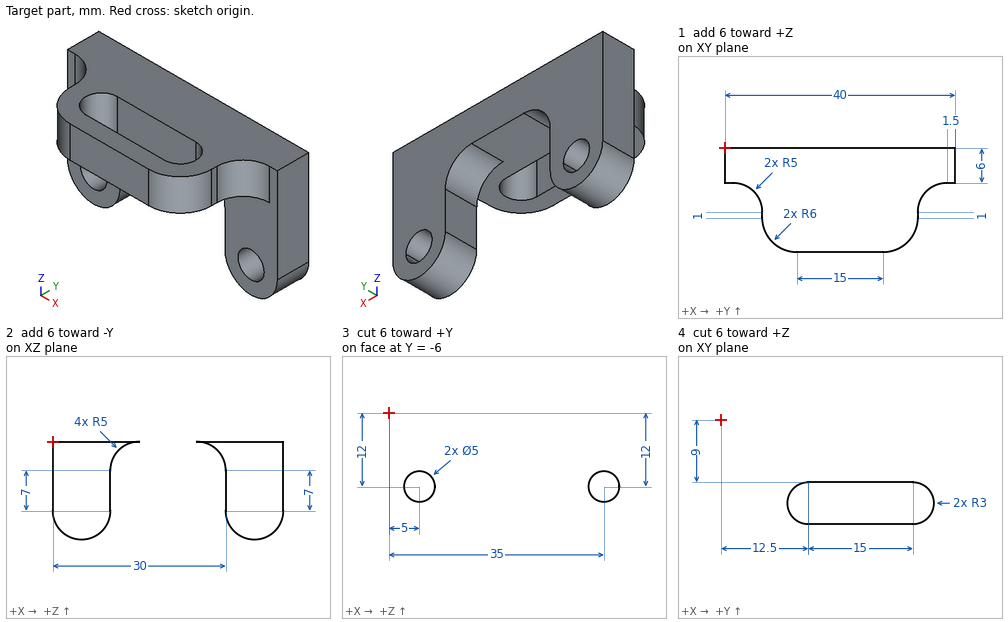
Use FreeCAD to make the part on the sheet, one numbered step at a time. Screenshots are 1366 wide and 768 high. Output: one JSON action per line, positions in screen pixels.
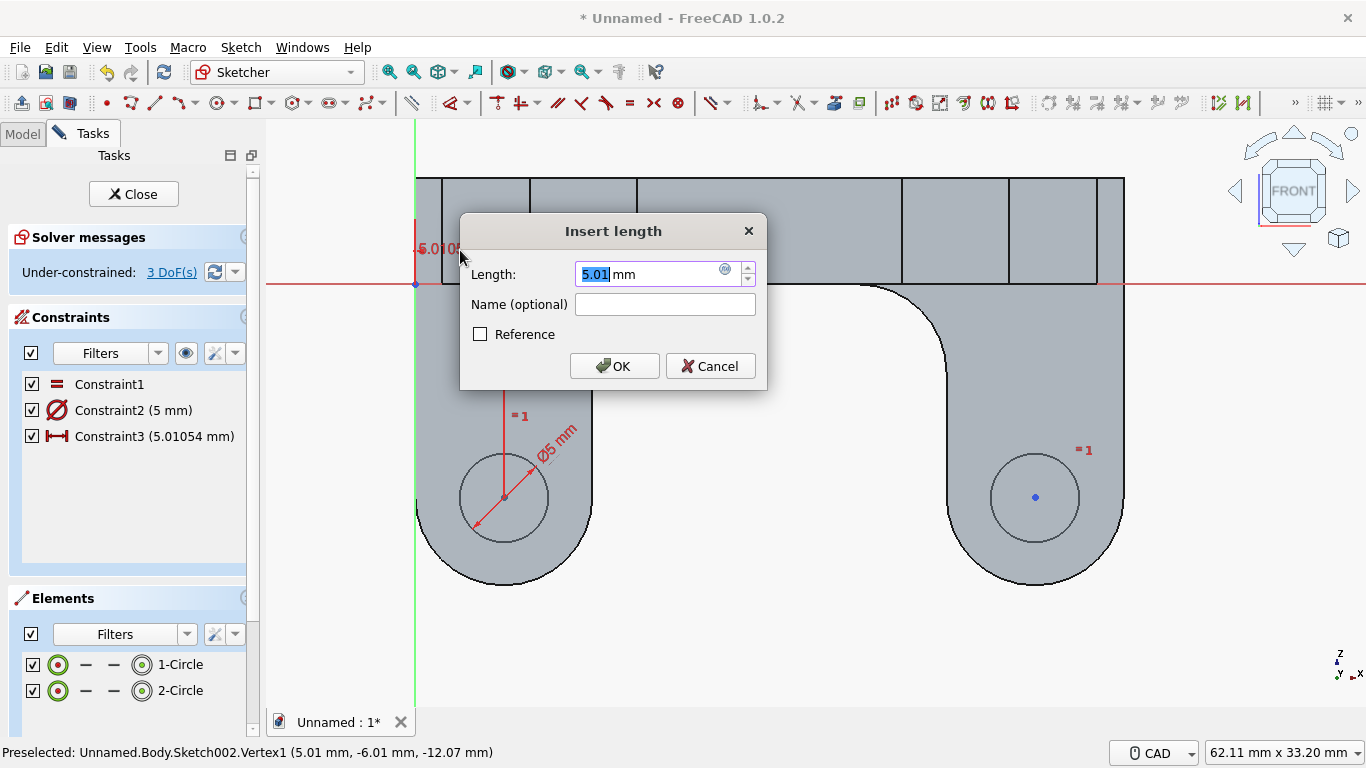
{"action": "type", "text": "5"}
{"action": "key", "text": "Return"}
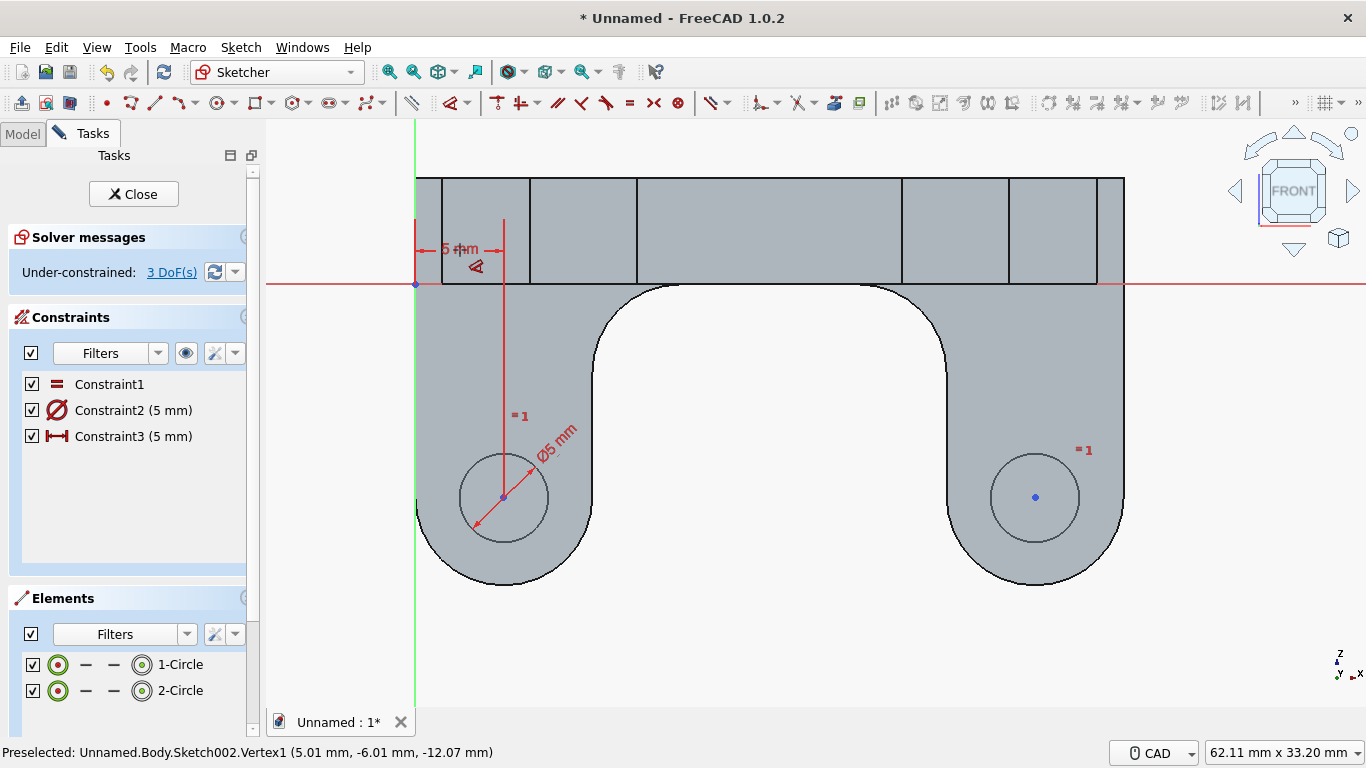
{"action": "left_click", "coordinate": [504, 498]}
{"action": "left_click", "coordinate": [381, 391]}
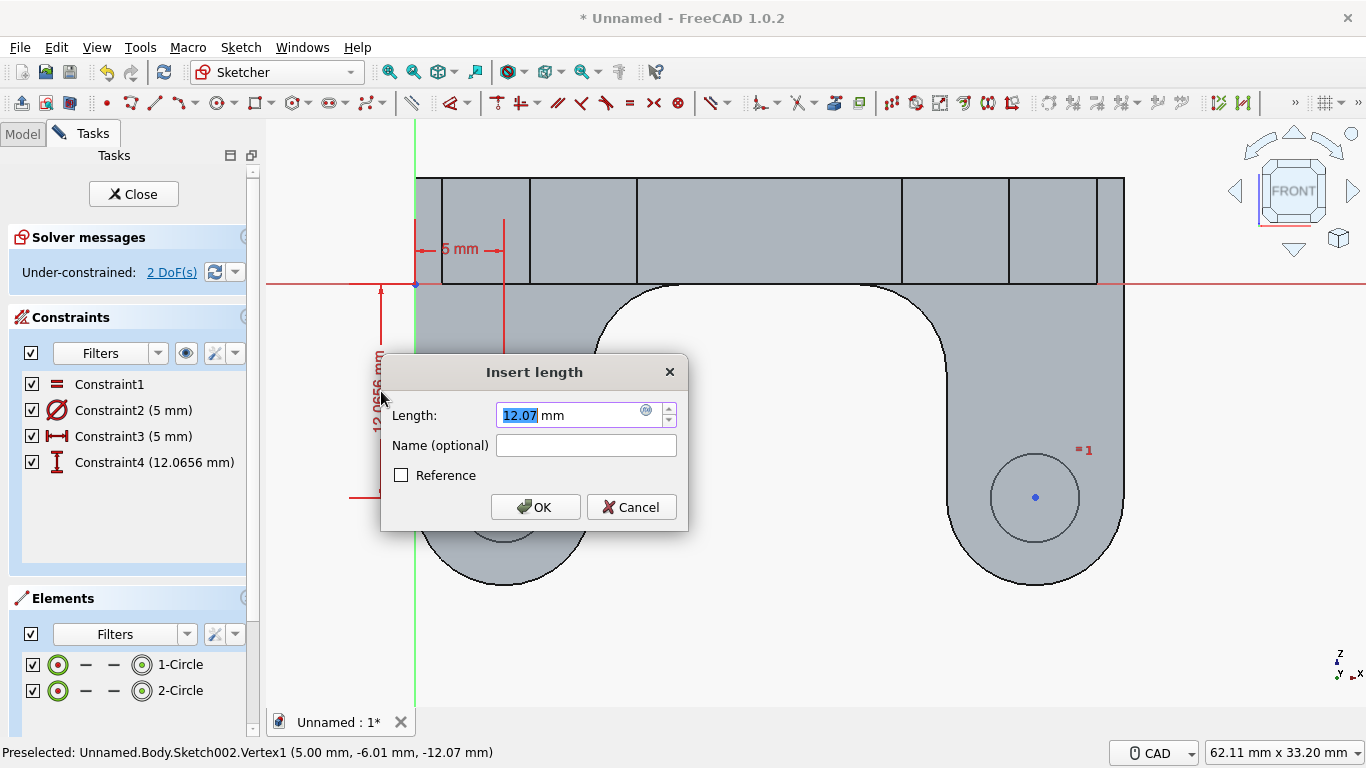
{"action": "type", "text": "12"}
{"action": "key", "text": "Return"}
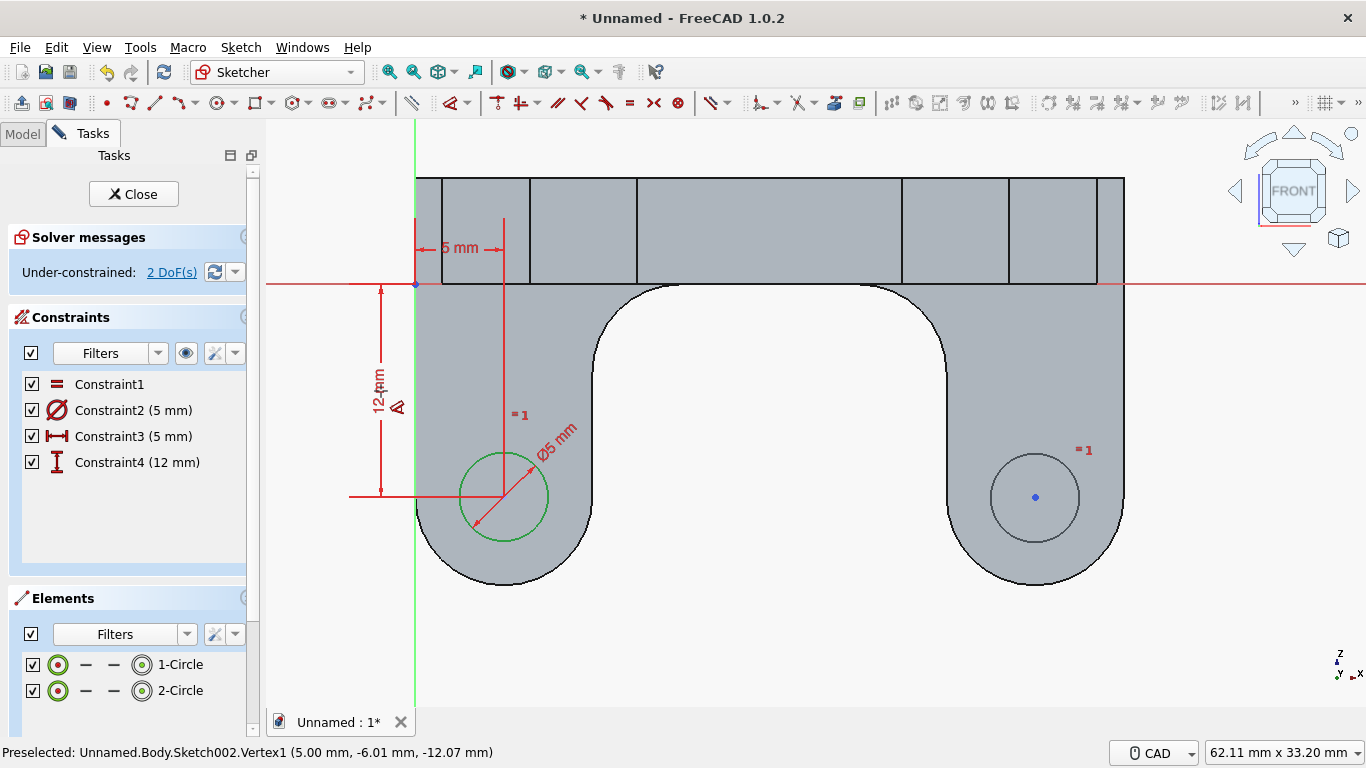
{"action": "left_click", "coordinate": [1035, 498]}
{"action": "left_click", "coordinate": [725, 250]}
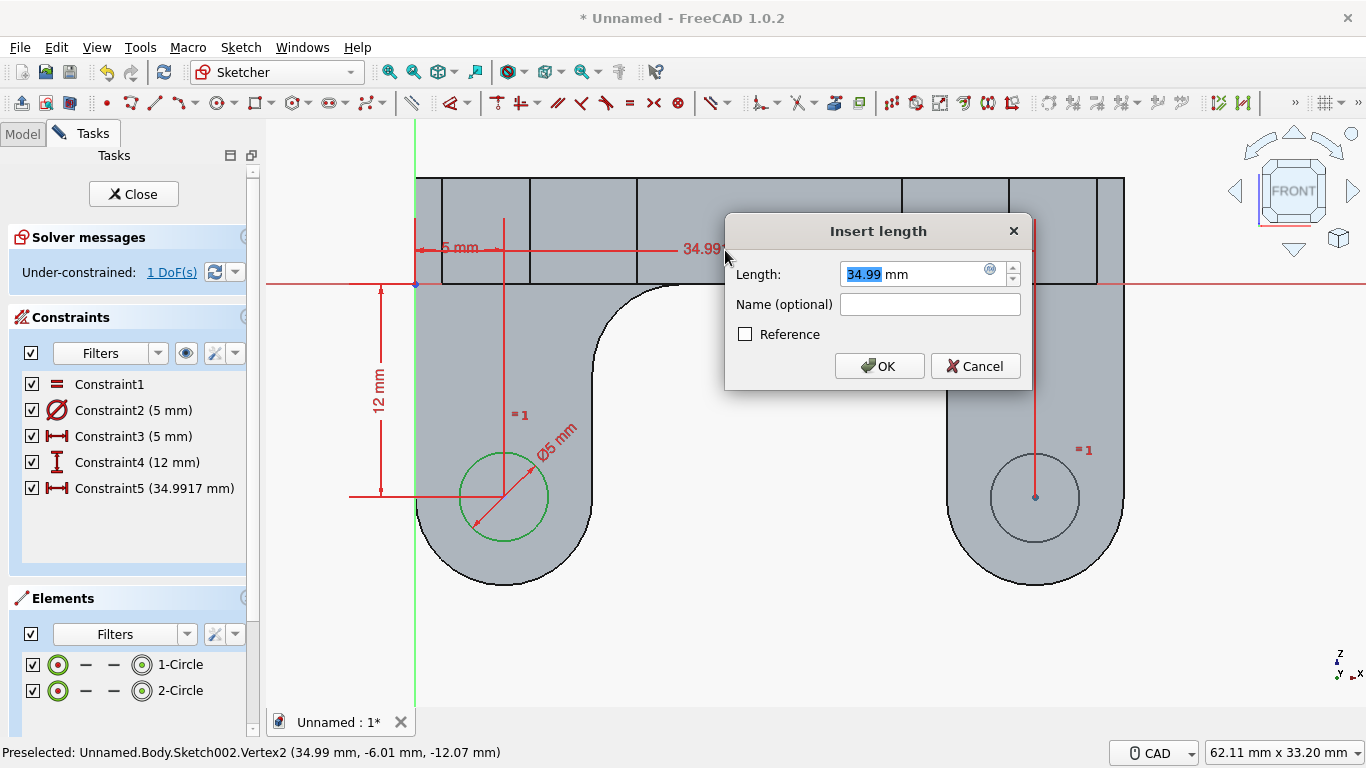
{"action": "type", "text": "35"}
{"action": "key", "text": "Return"}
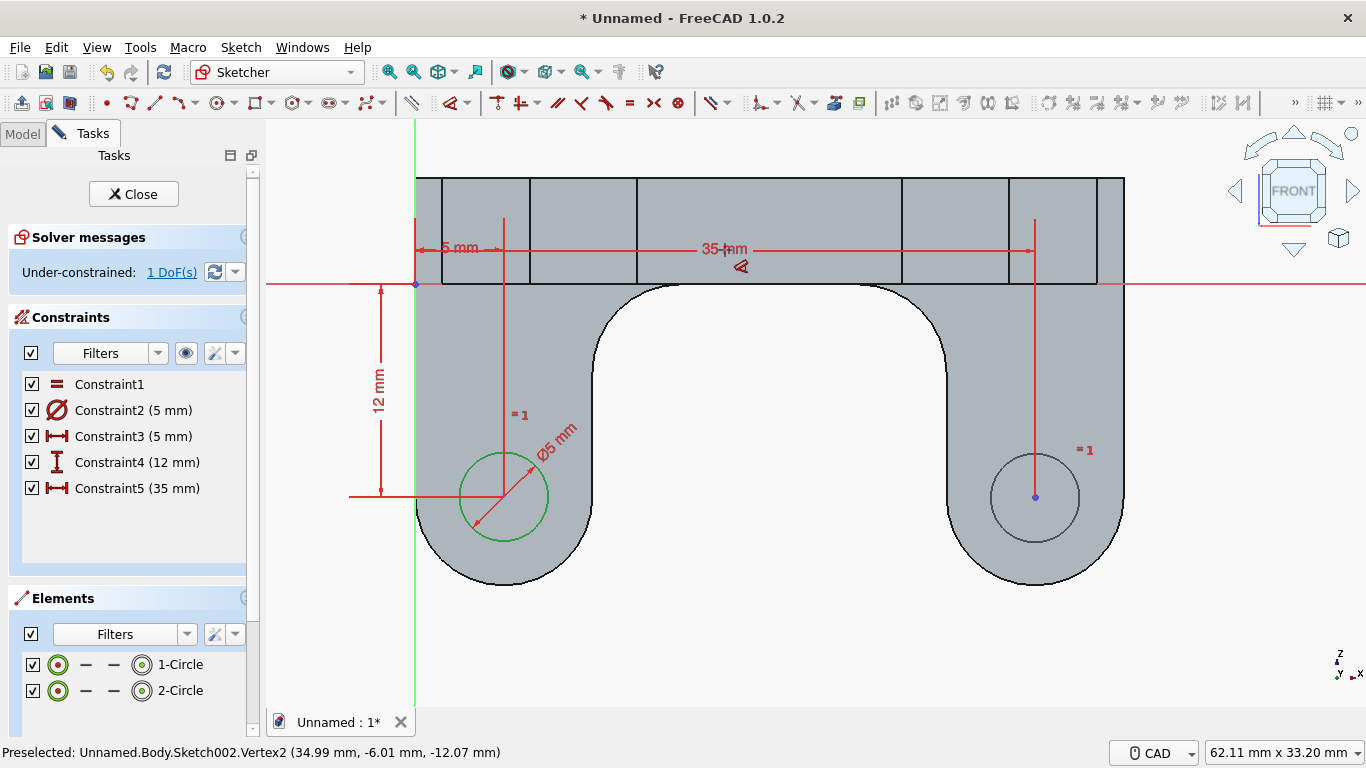
{"action": "left_click", "coordinate": [1035, 498]}
{"action": "left_click", "coordinate": [381, 342]}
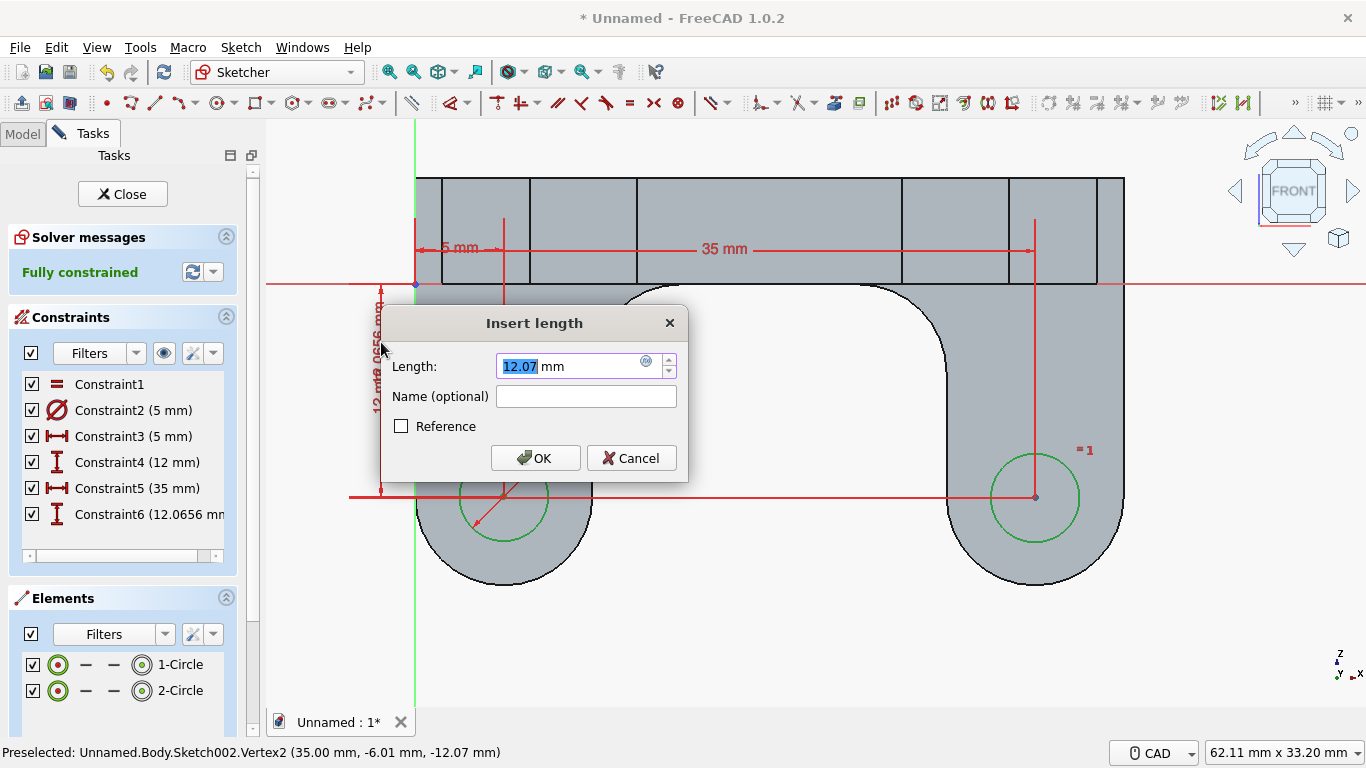
{"action": "type", "text": "12"}
{"action": "key", "text": "Return"}
{"action": "key", "text": "Escape"}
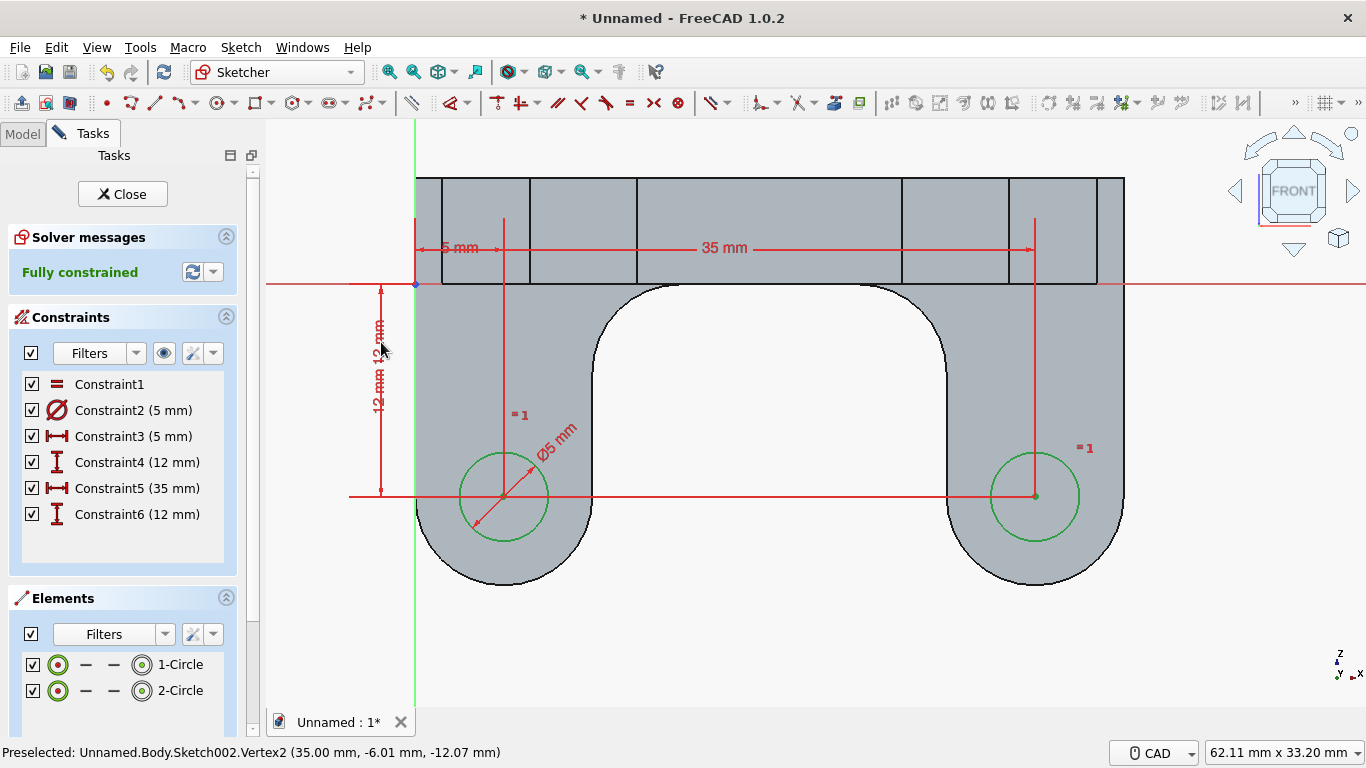
{"action": "left_click", "coordinate": [123, 194]}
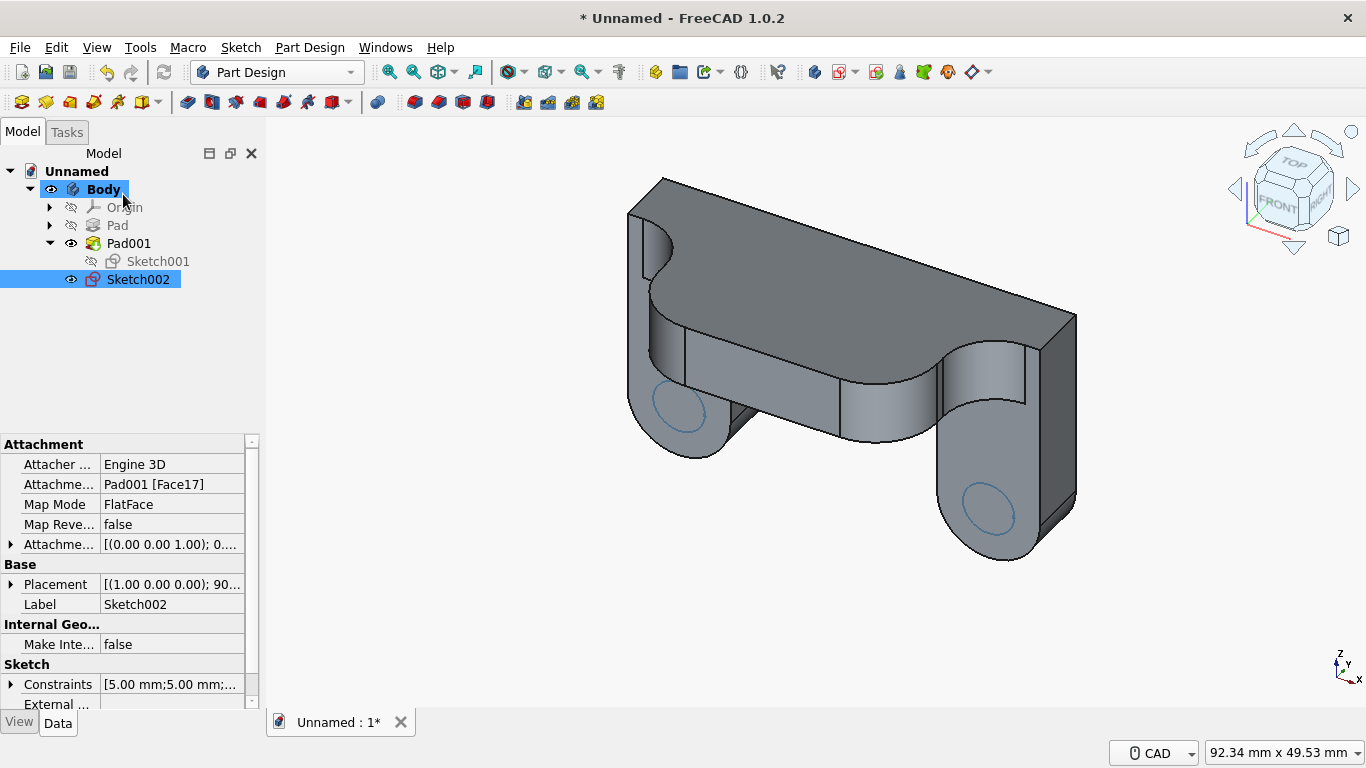
{"action": "left_click", "coordinate": [188, 102]}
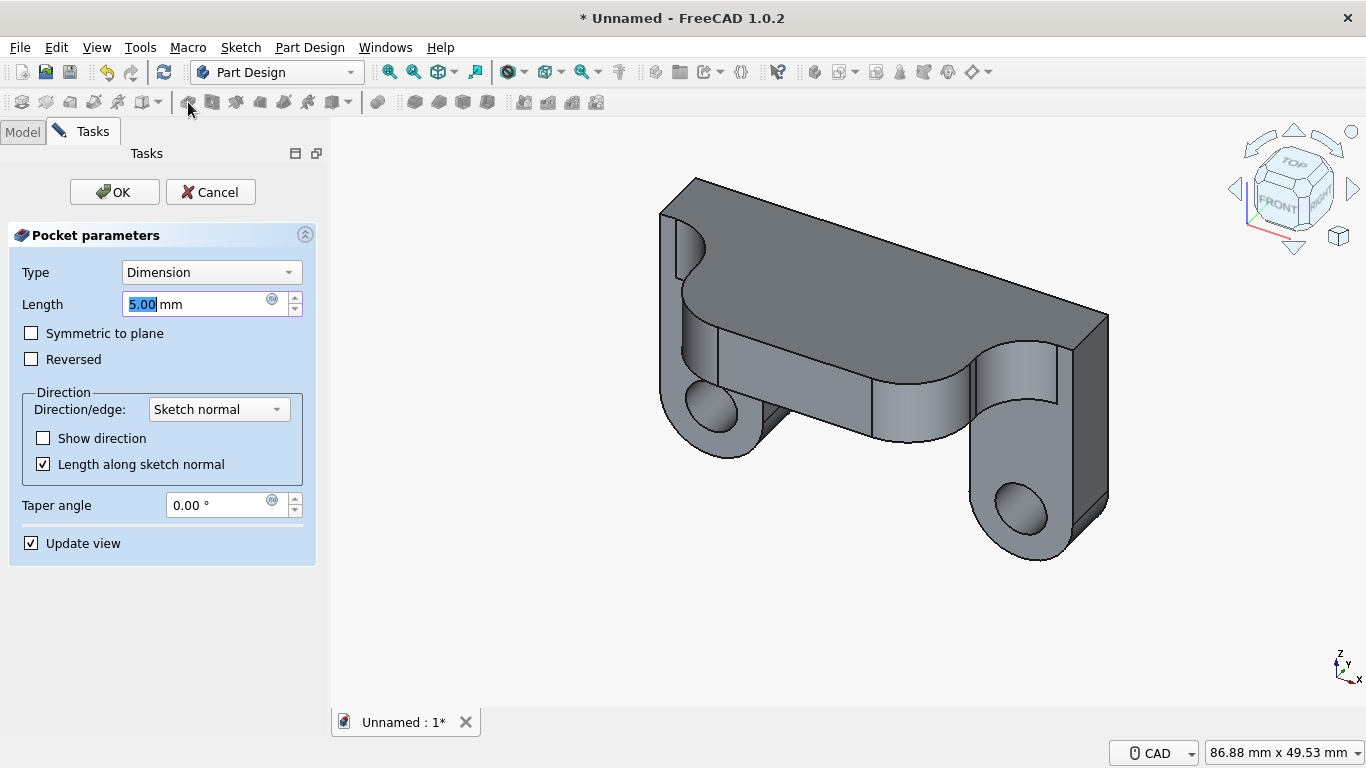
{"action": "type", "text": "6"}
{"action": "key", "text": "Tab"}